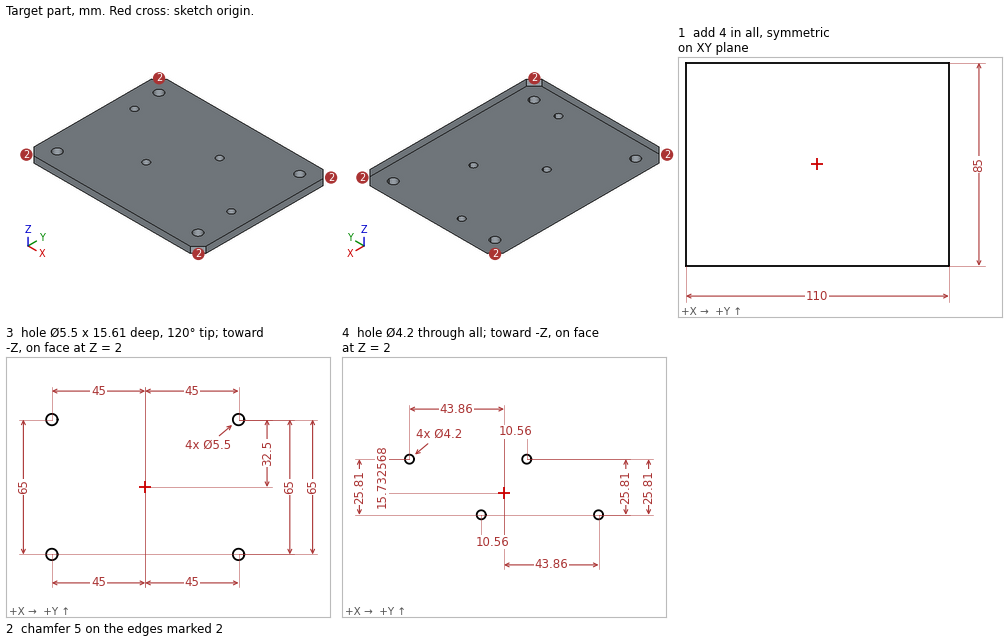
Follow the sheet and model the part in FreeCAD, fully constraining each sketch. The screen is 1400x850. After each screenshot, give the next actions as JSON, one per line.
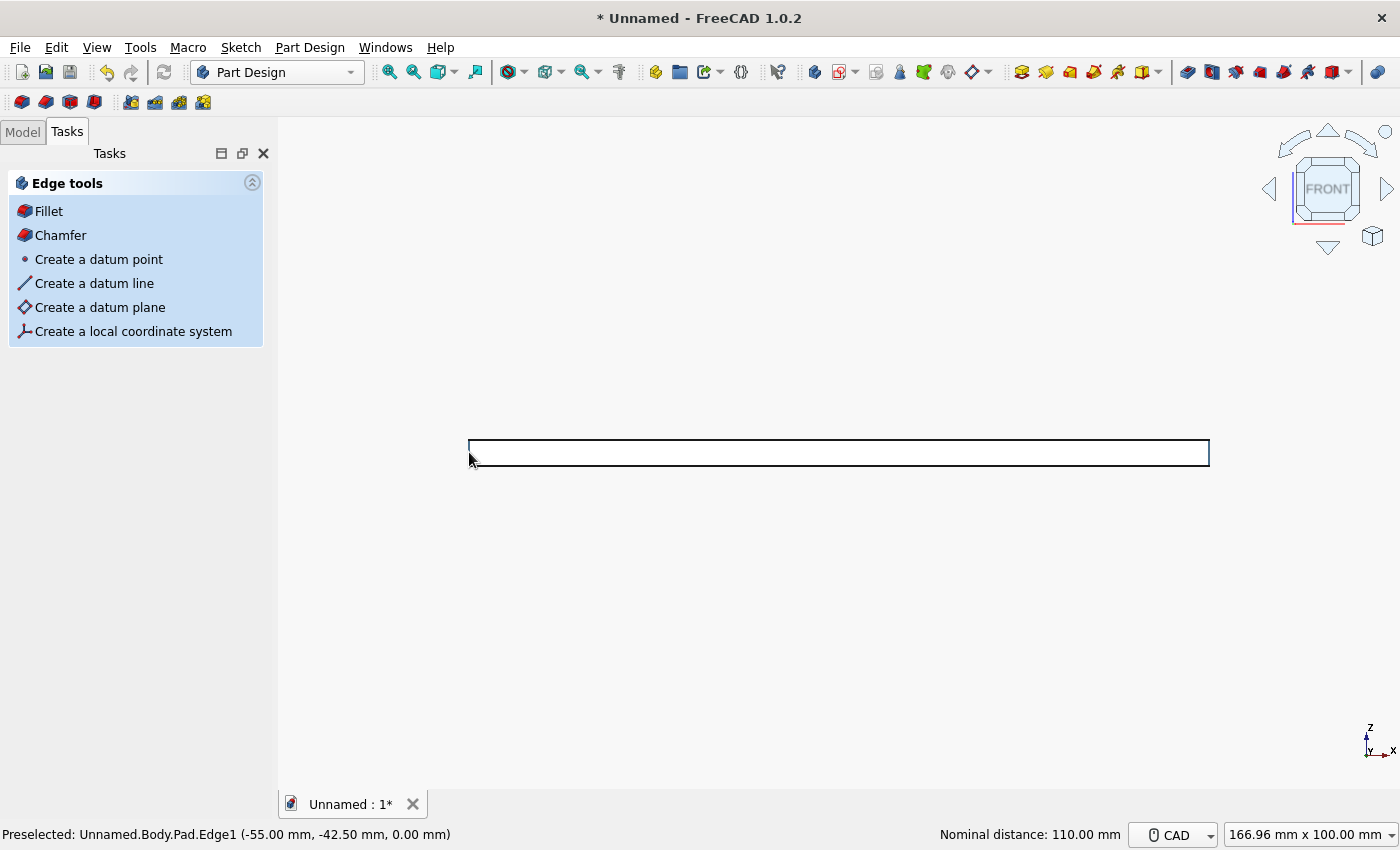
{"action": "key", "text": "3"}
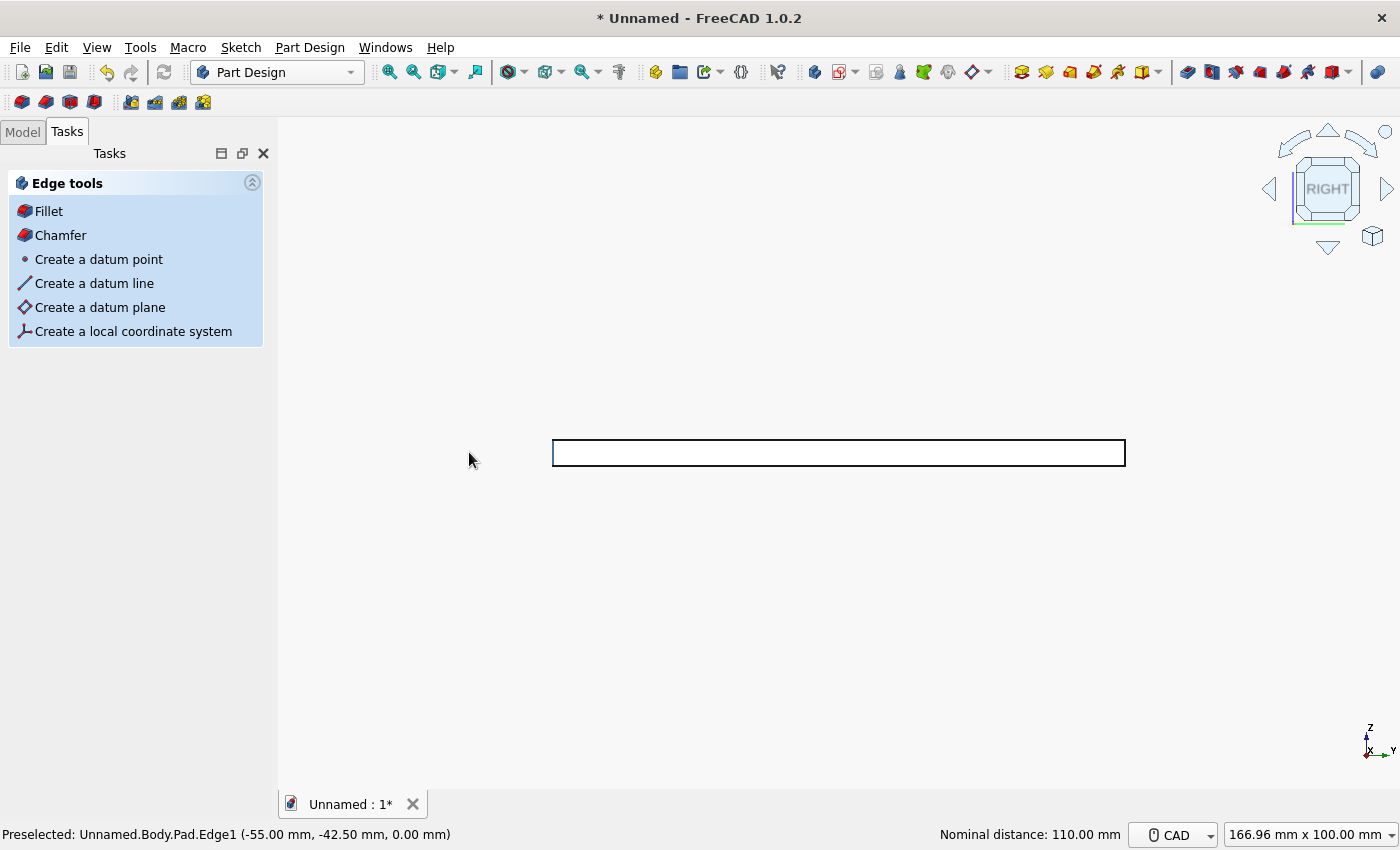
{"action": "left_click", "coordinate": [1125, 452], "text": "ctrl"}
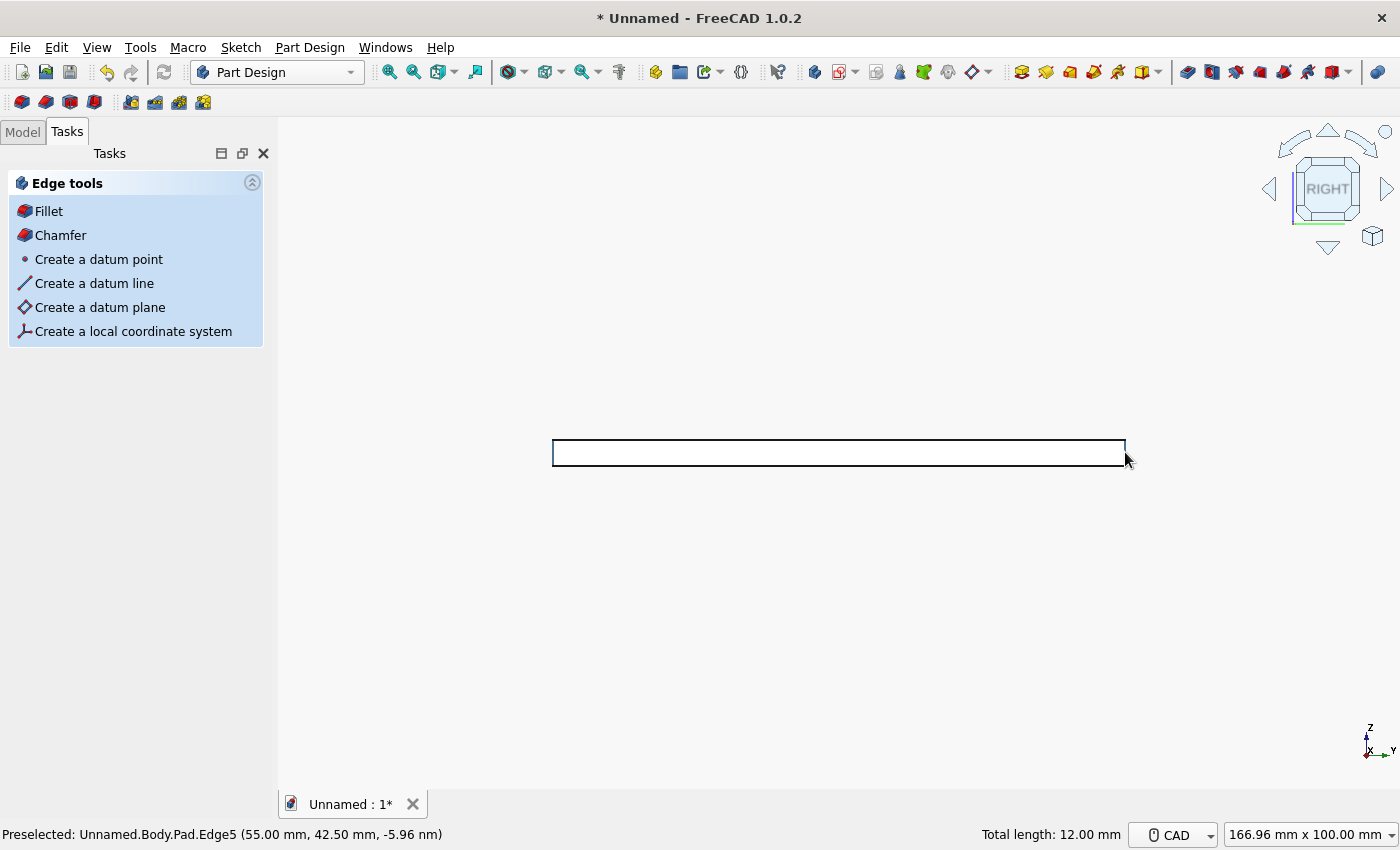
{"action": "key", "text": "5"}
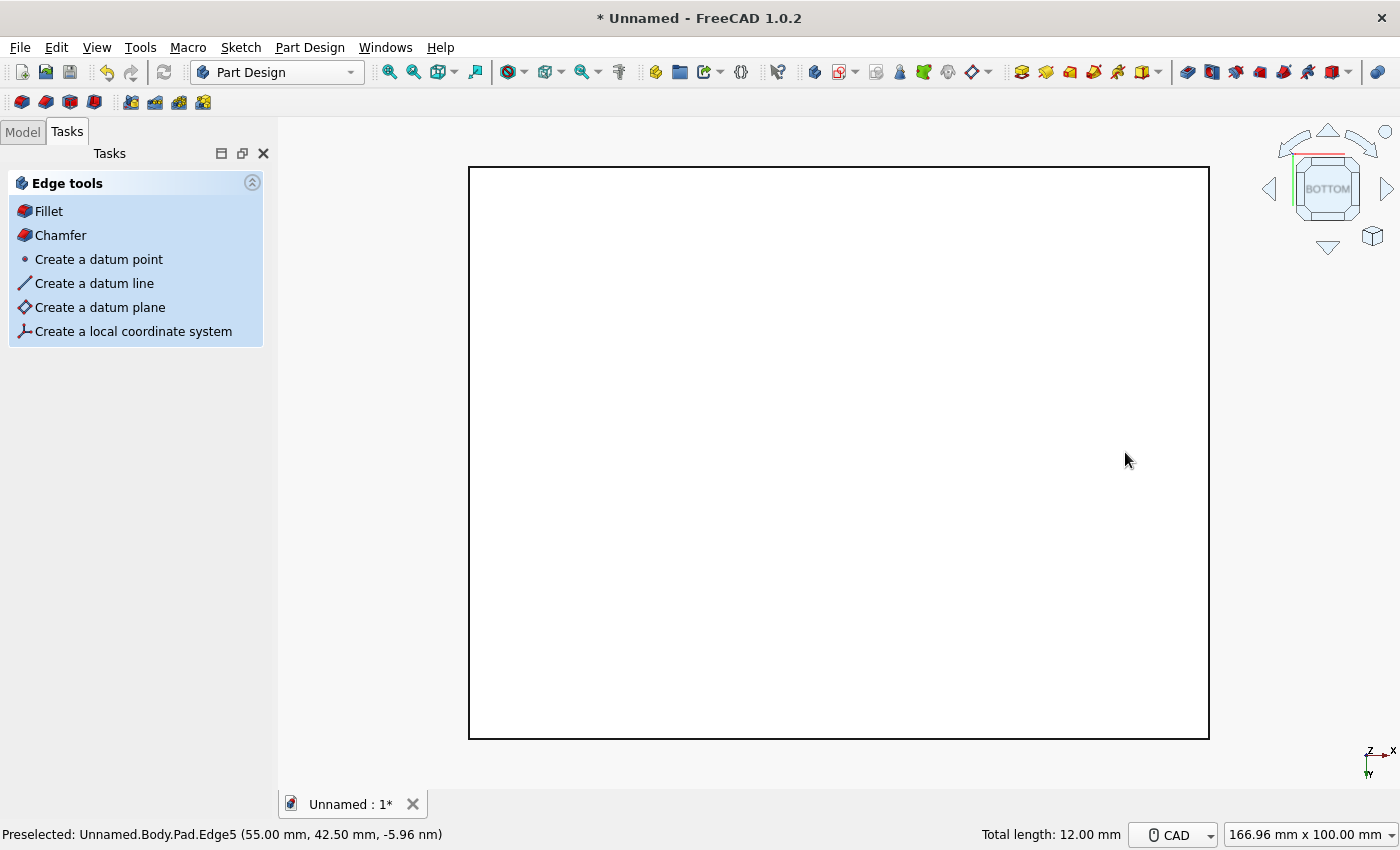
{"action": "key", "text": "4"}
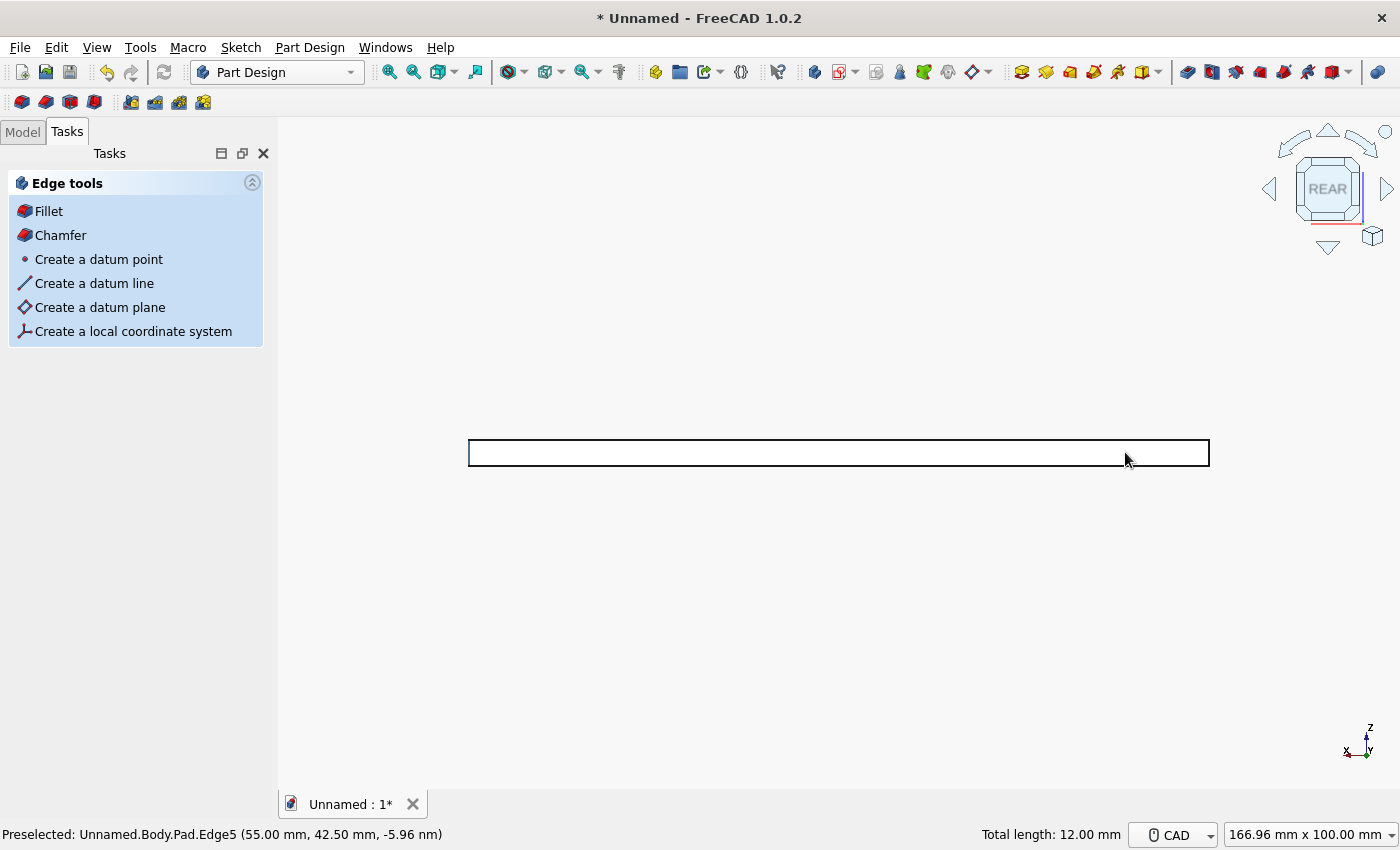
{"action": "left_click", "coordinate": [1209, 452], "text": "ctrl"}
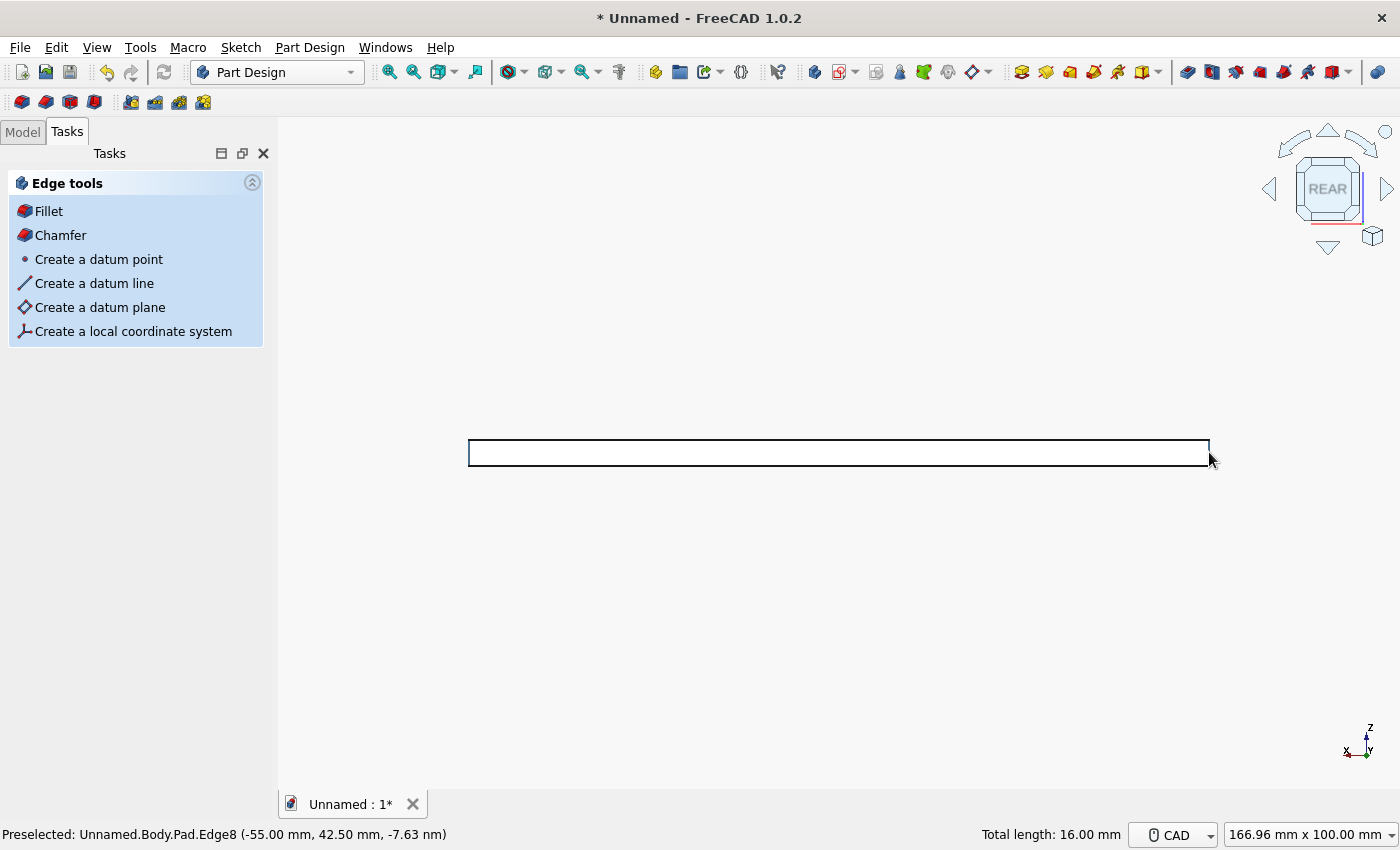
{"action": "left_click", "coordinate": [46, 102]}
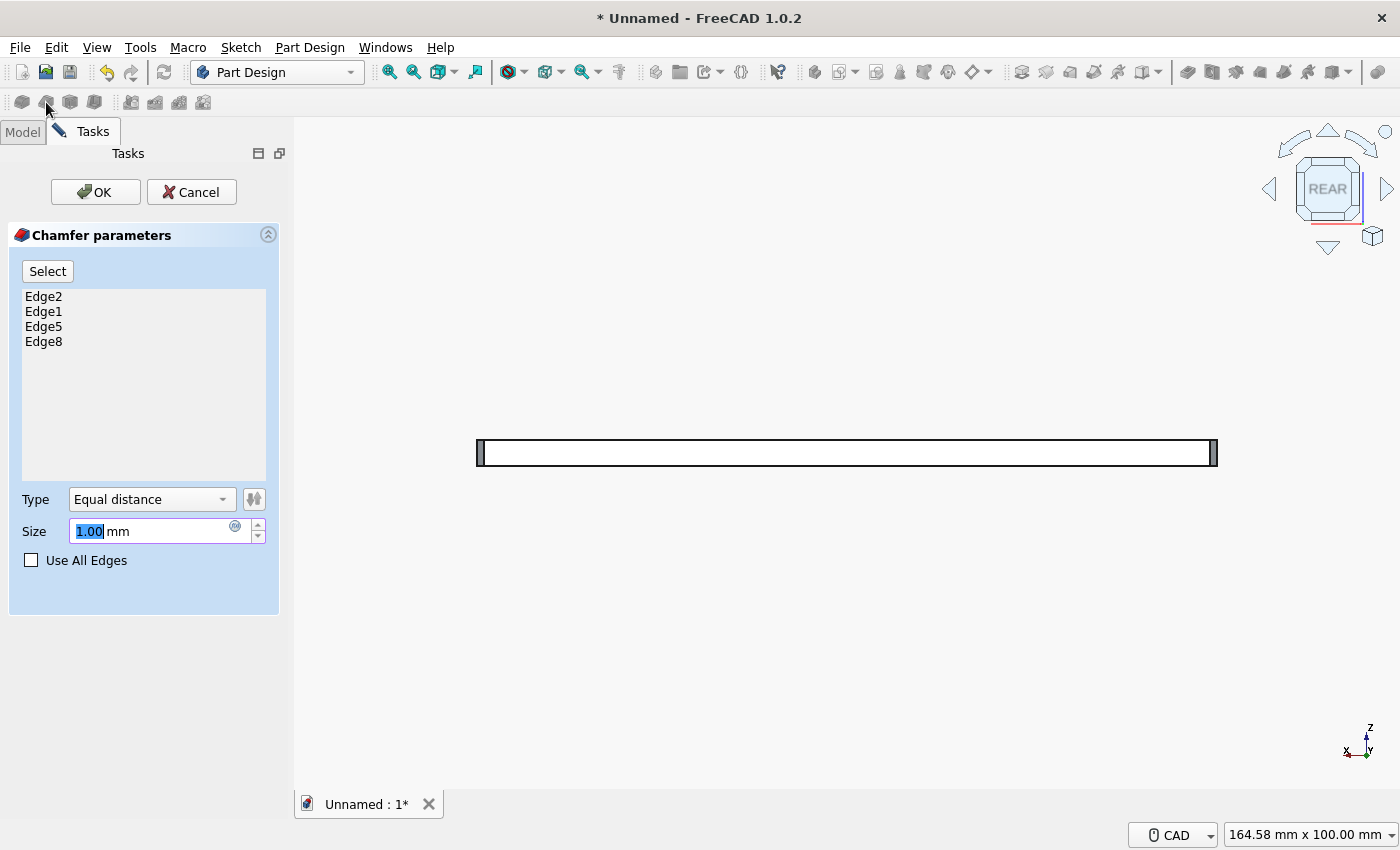
{"action": "type", "text": "5"}
{"action": "key", "text": "Tab"}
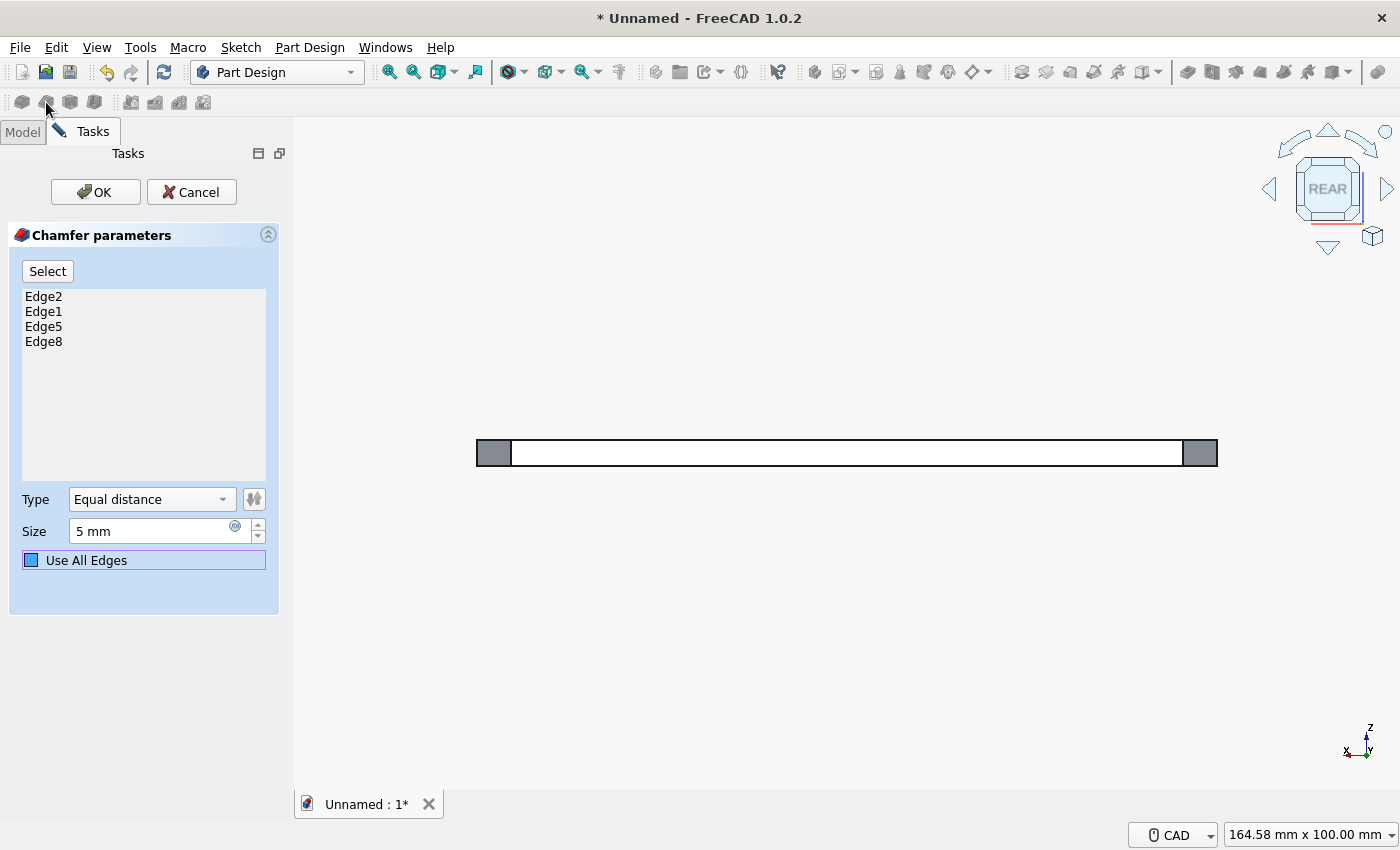
{"action": "left_click", "coordinate": [96, 192]}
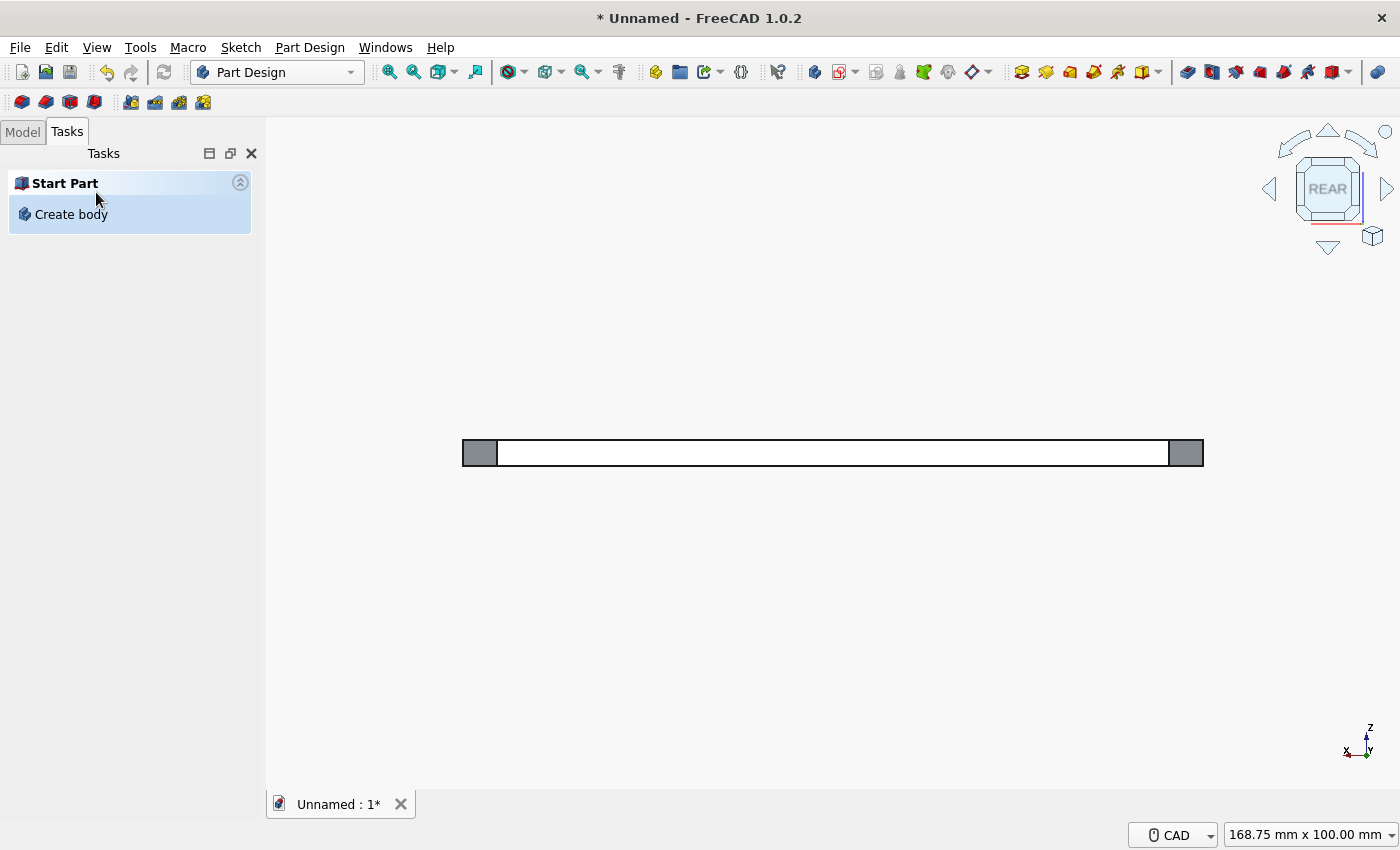
{"action": "key", "text": "0"}